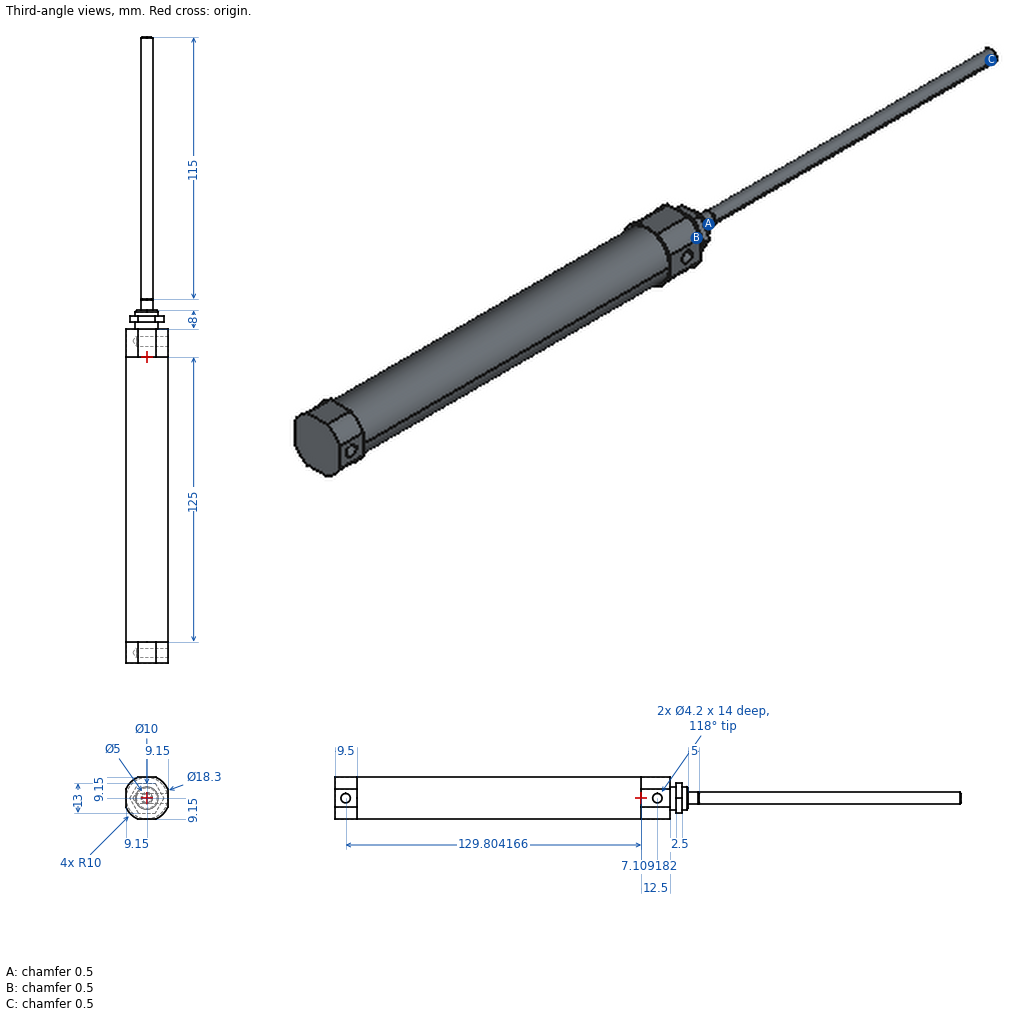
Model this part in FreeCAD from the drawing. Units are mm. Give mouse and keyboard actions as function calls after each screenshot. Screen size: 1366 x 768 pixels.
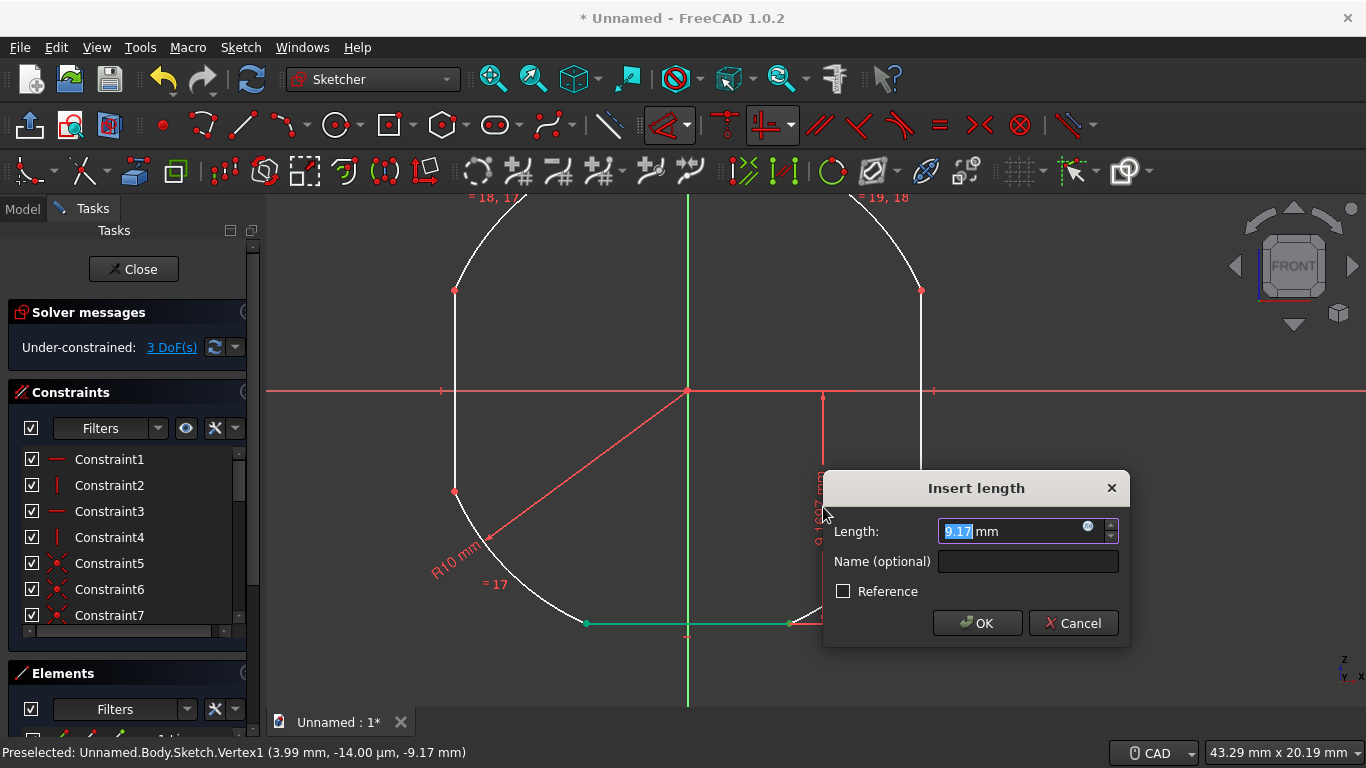
text(9.15)
key(Return)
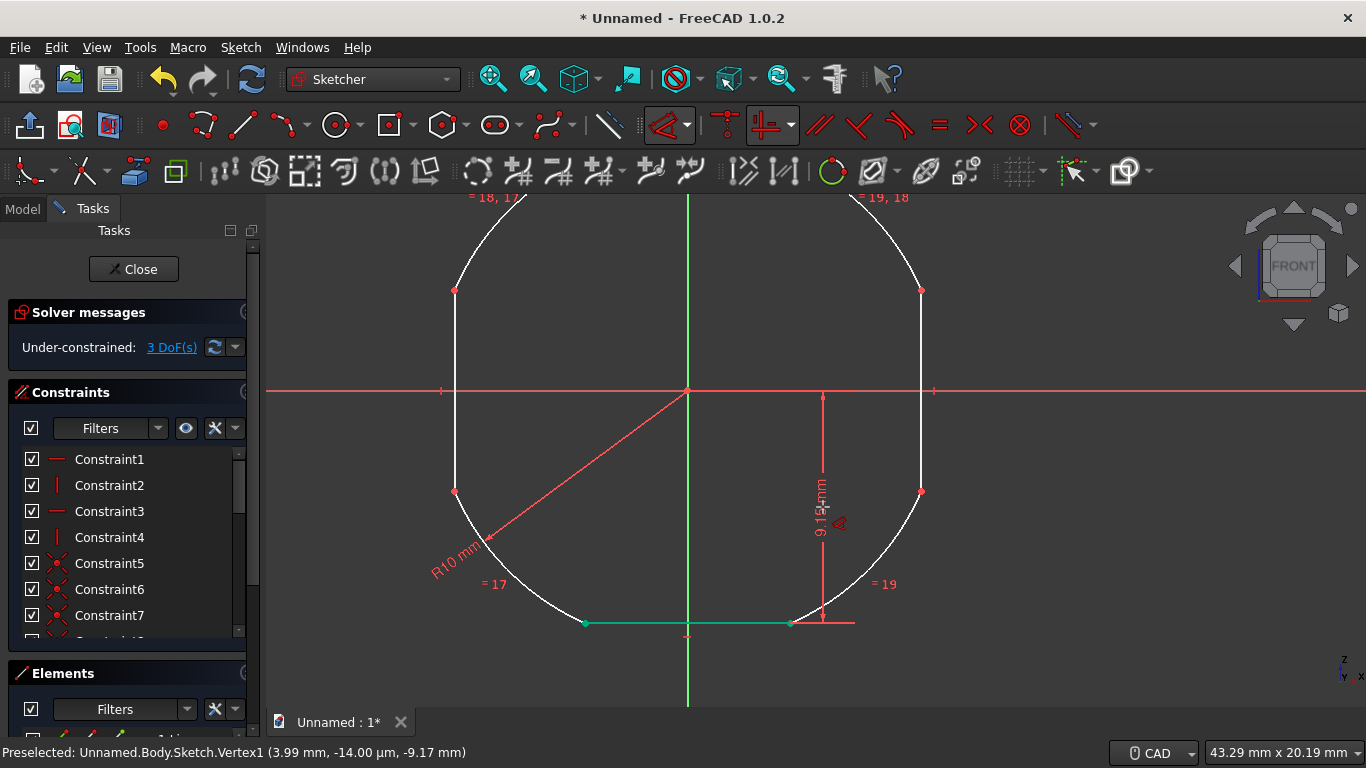
click(455, 491)
click(571, 525)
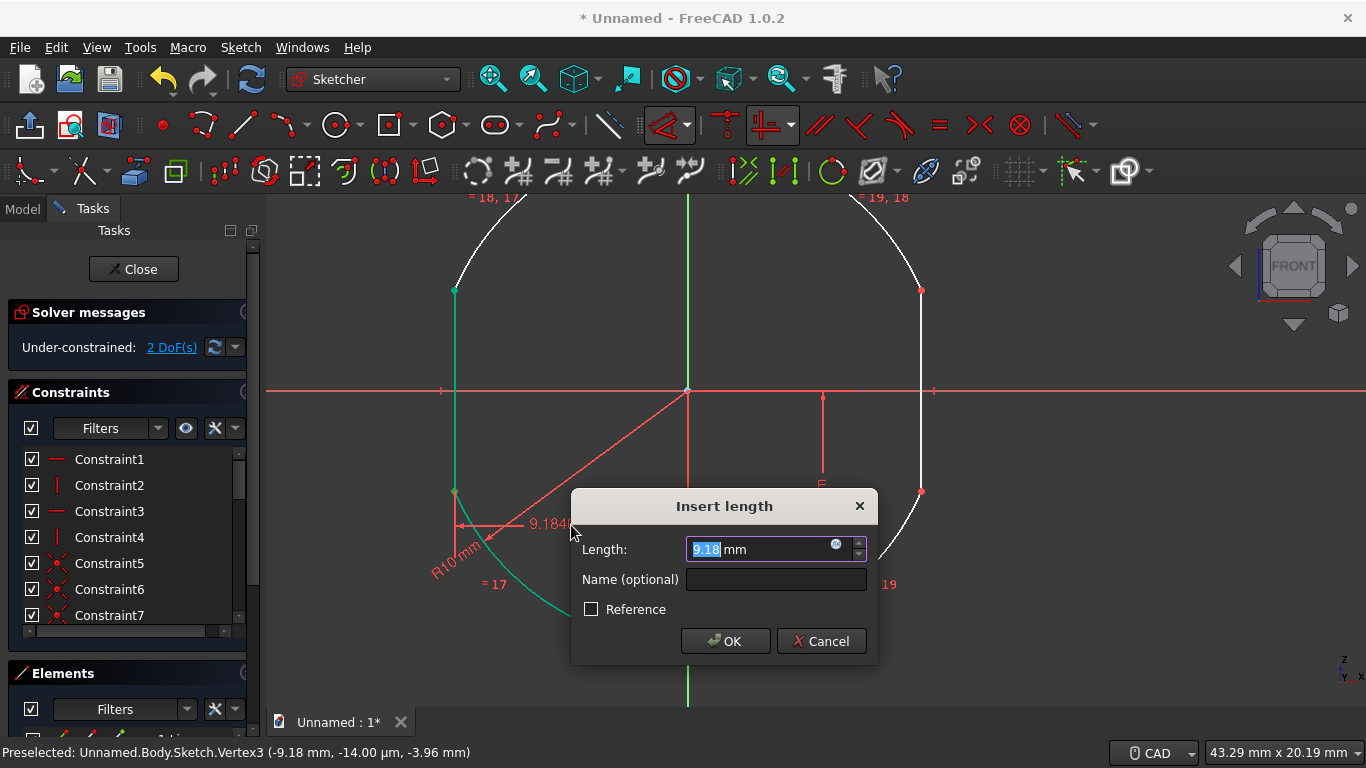
text(9.15)
key(Return)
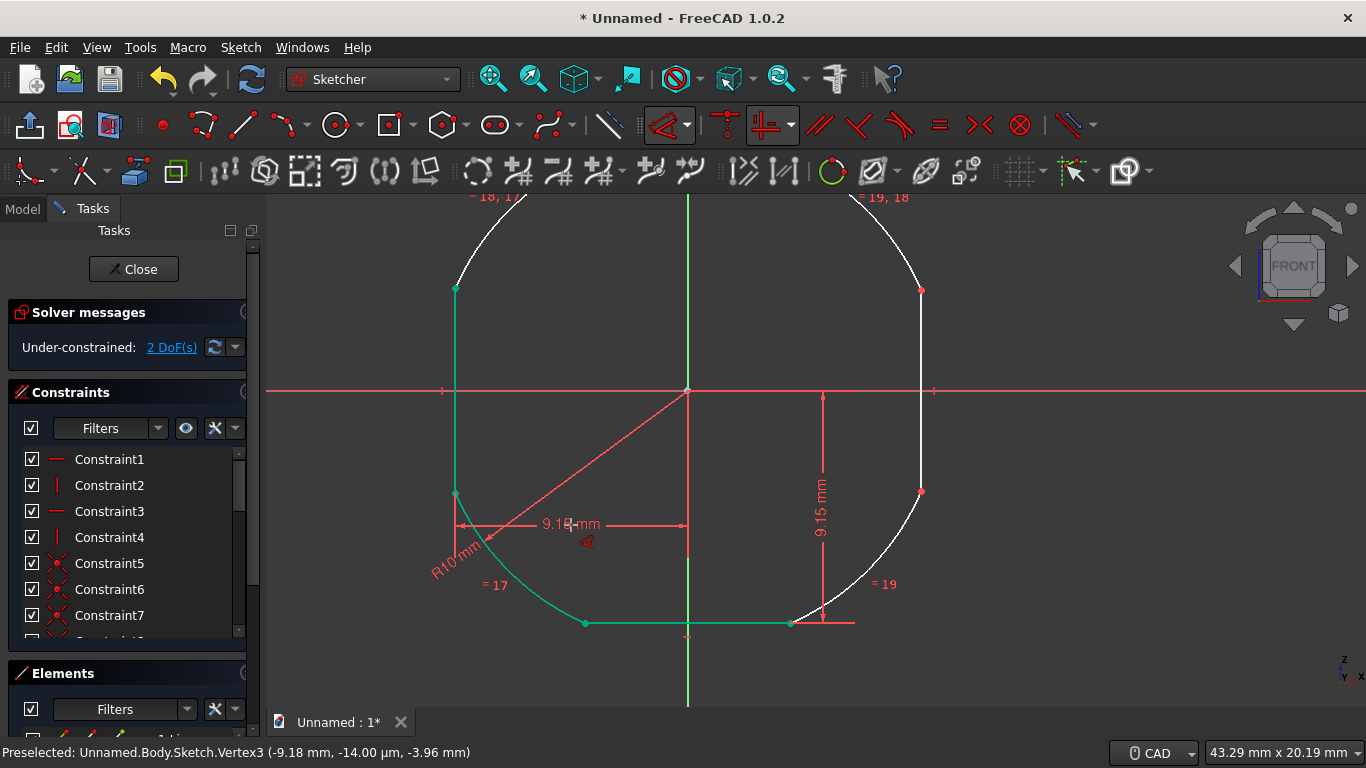
scroll(869, 572, down, 2)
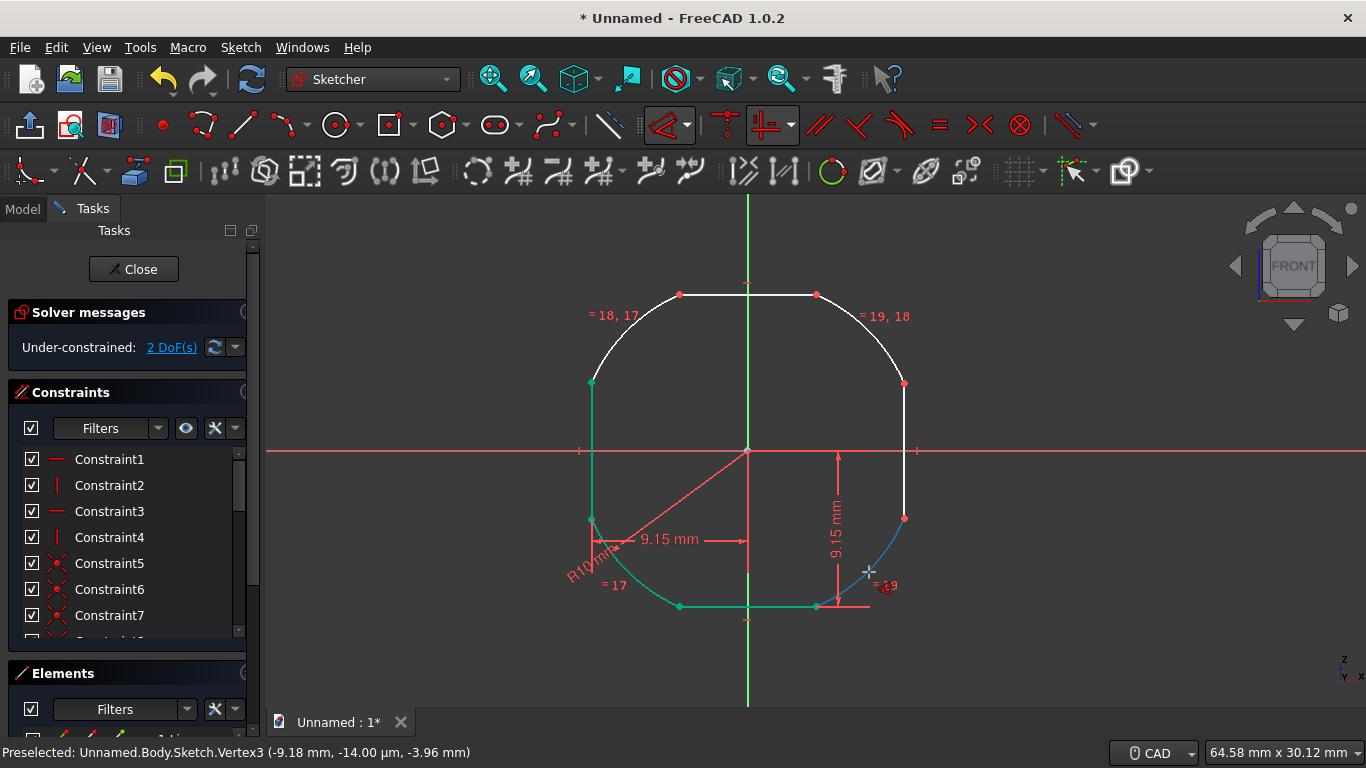
click(679, 295)
click(645, 373)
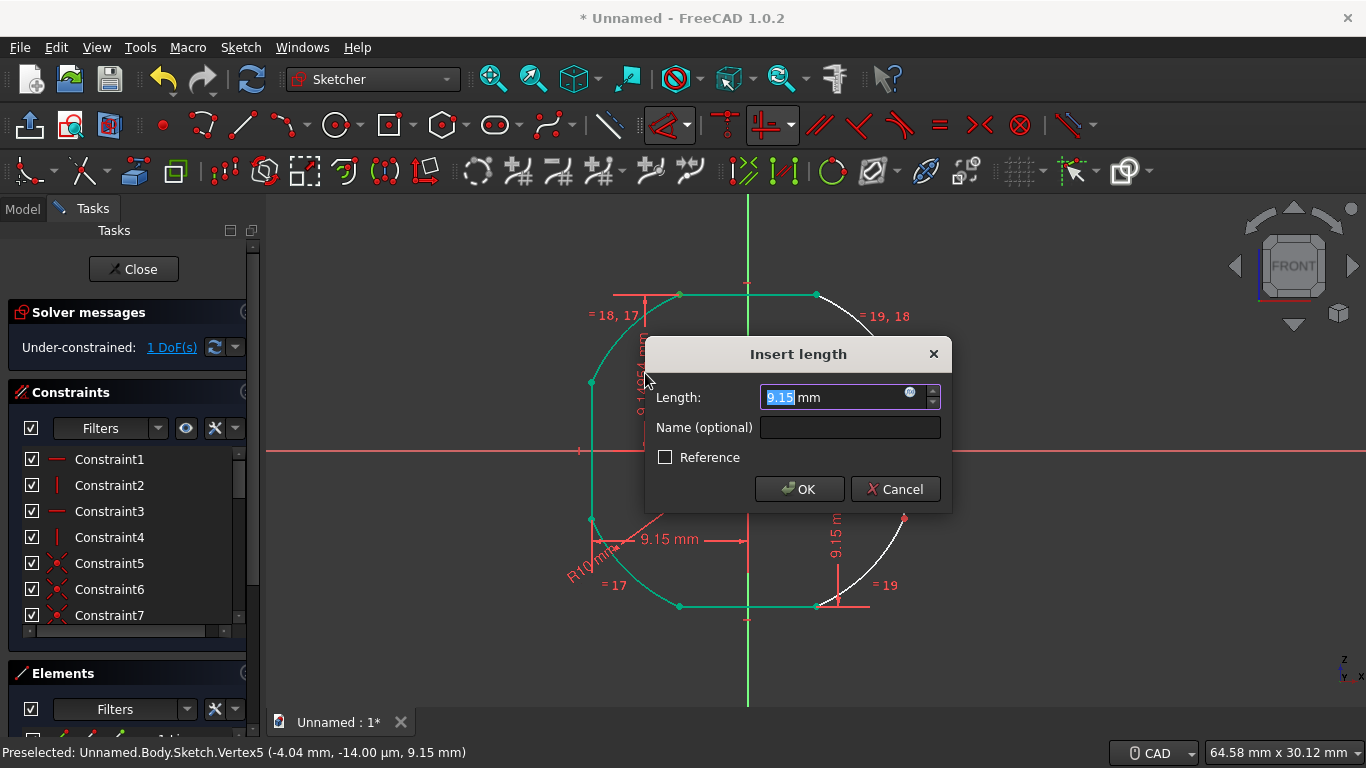
text(9.15)
key(Return)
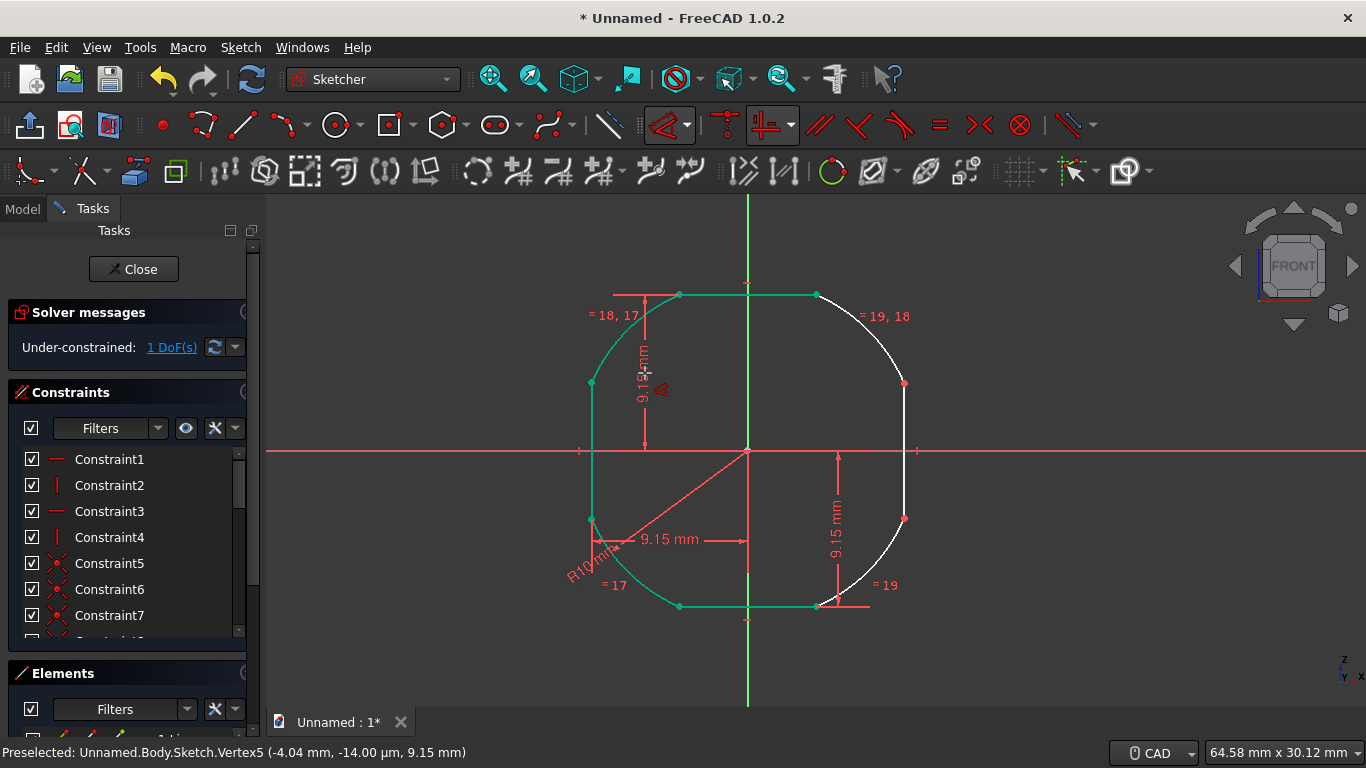
click(904, 383)
click(826, 349)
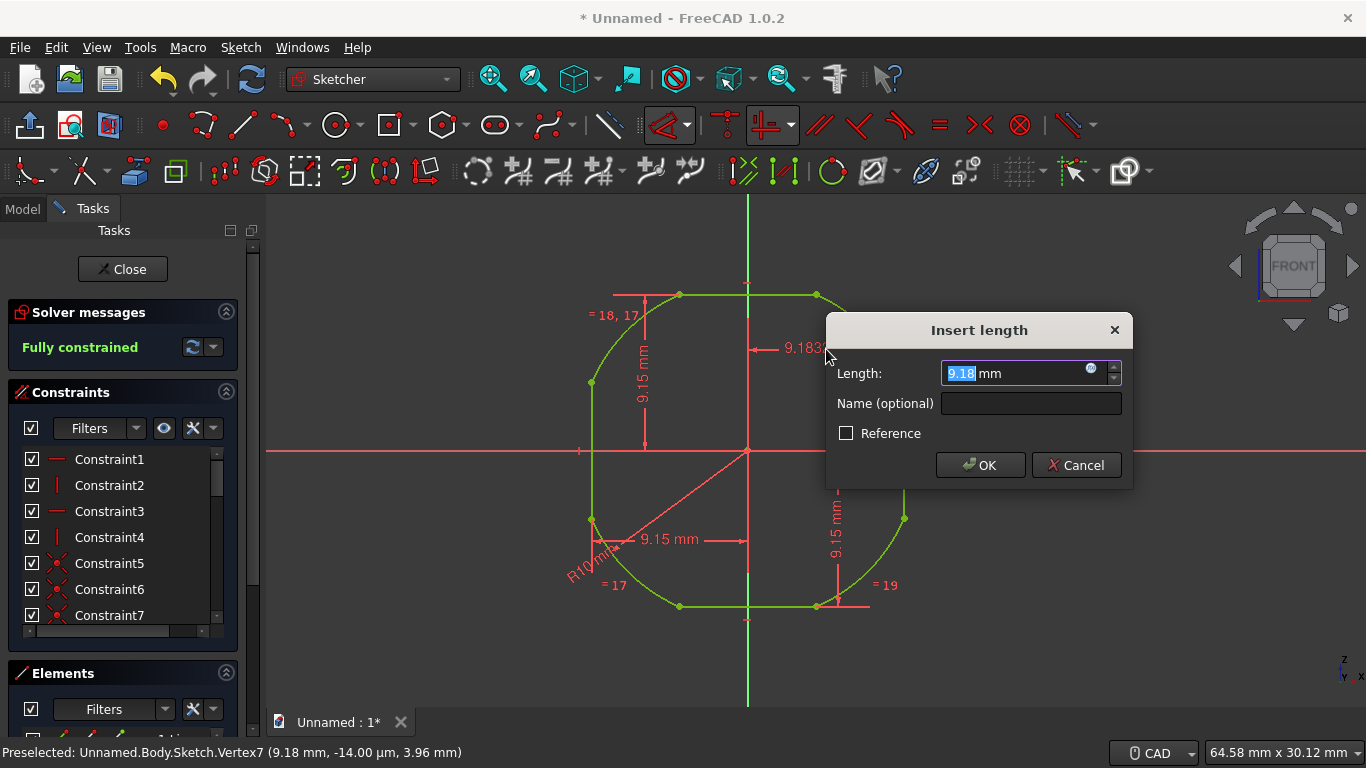
text(9.15)
key(Return)
key(Escape)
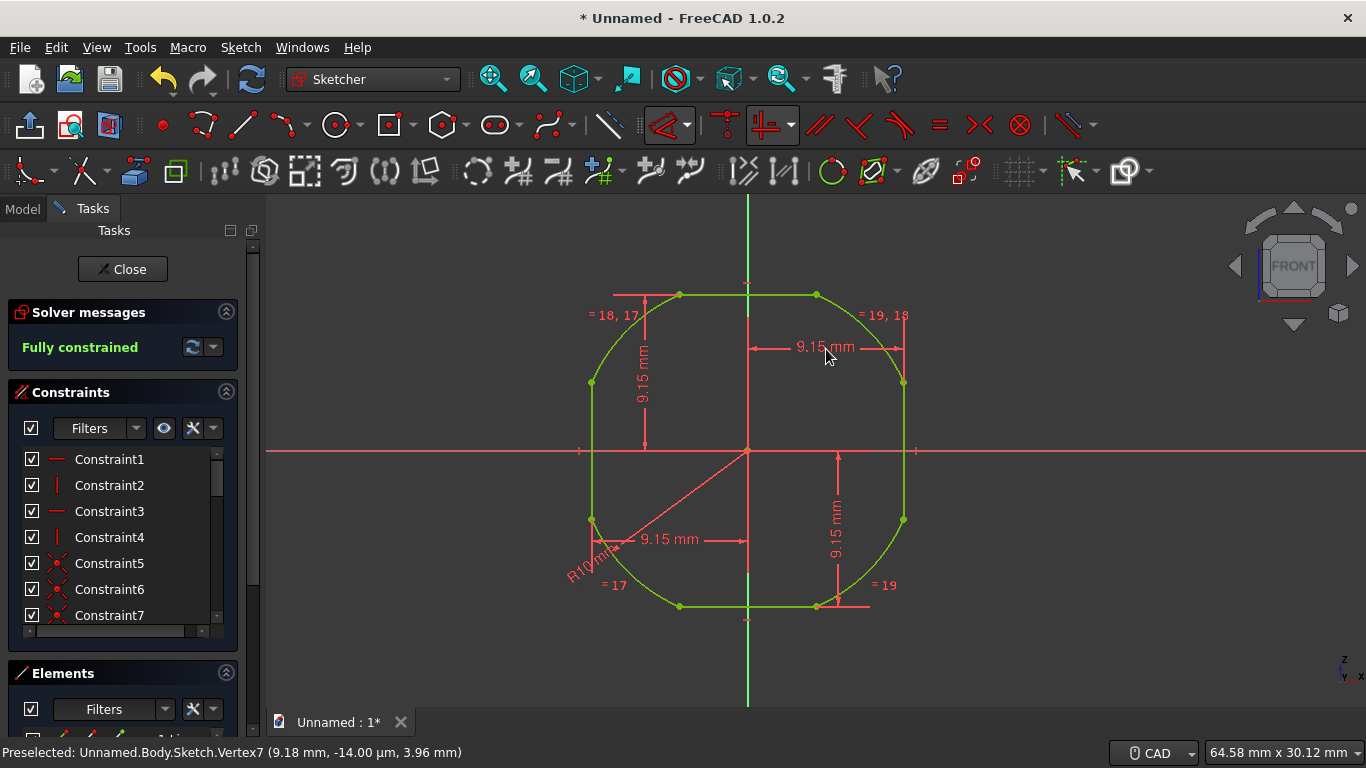
click(123, 269)